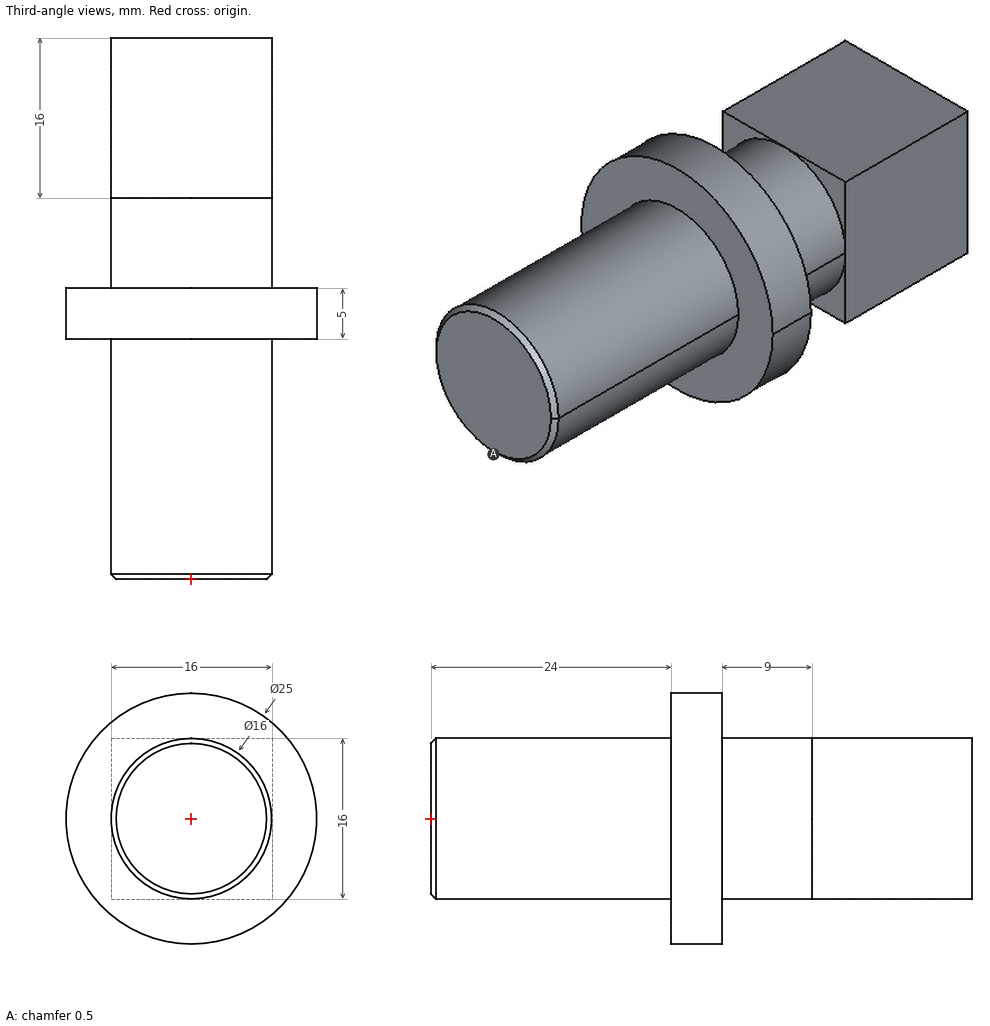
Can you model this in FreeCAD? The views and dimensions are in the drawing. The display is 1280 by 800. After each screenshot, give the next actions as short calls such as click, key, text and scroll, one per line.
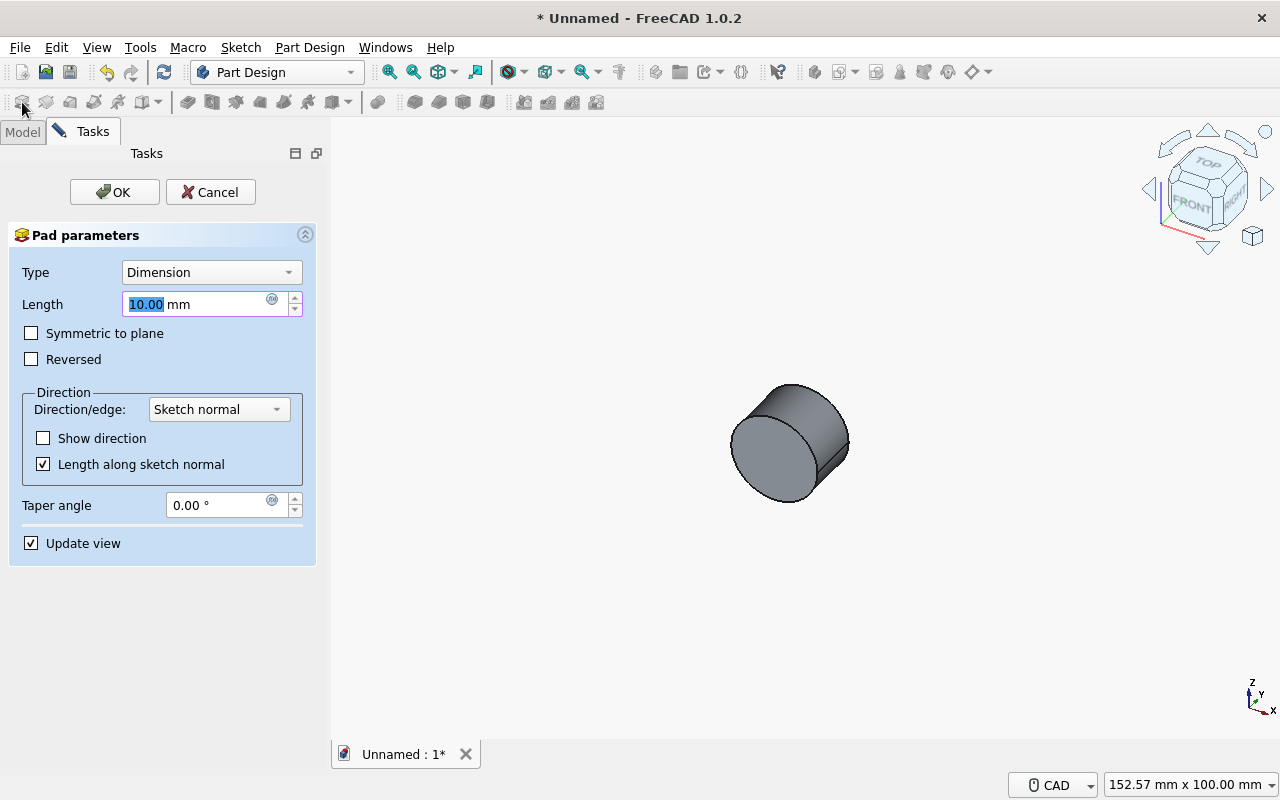
text(24)
key(Tab)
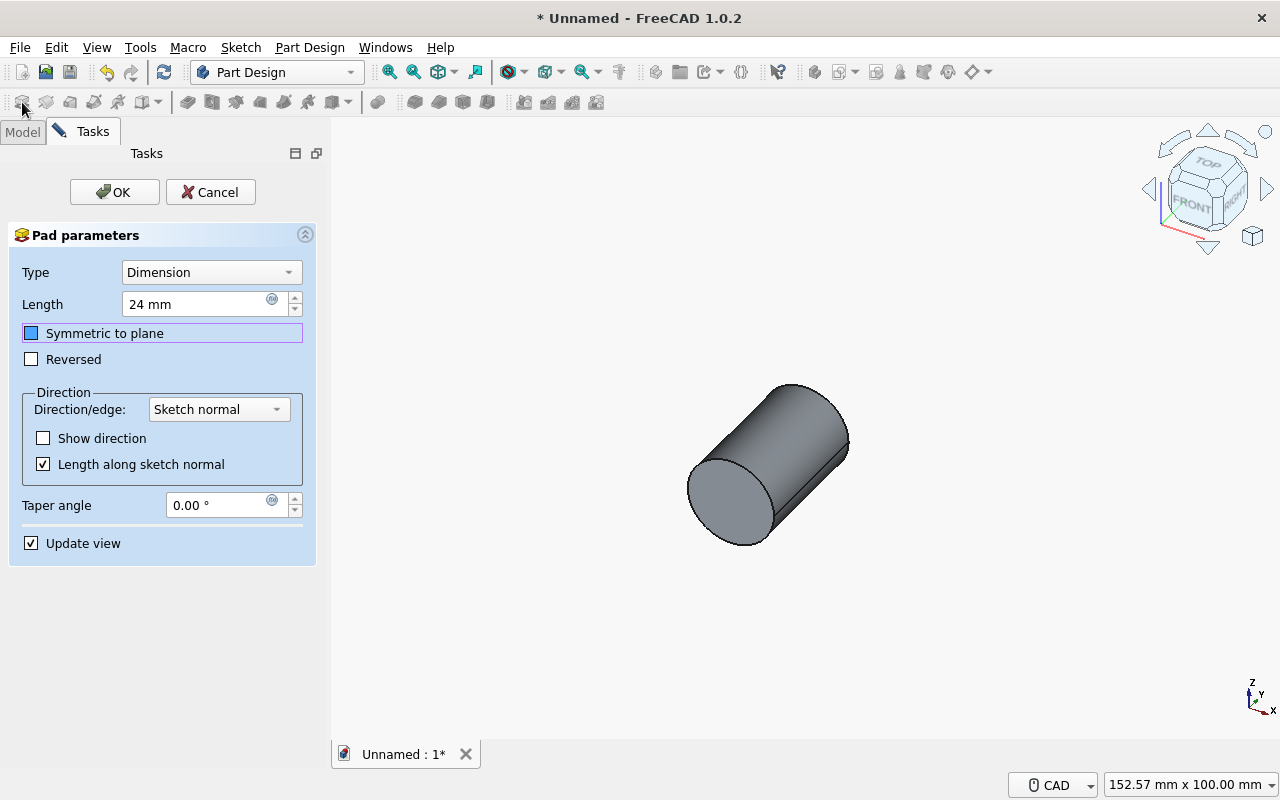
click(30, 359)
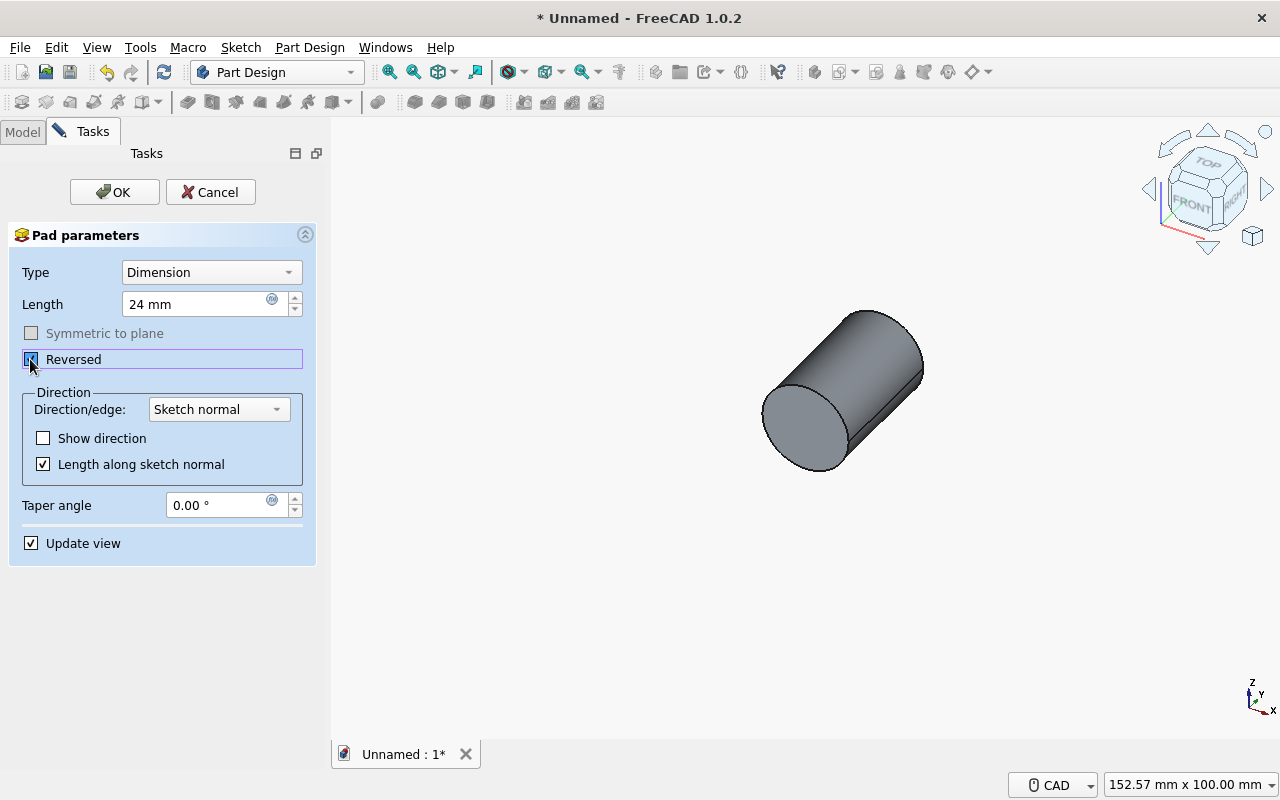
click(115, 192)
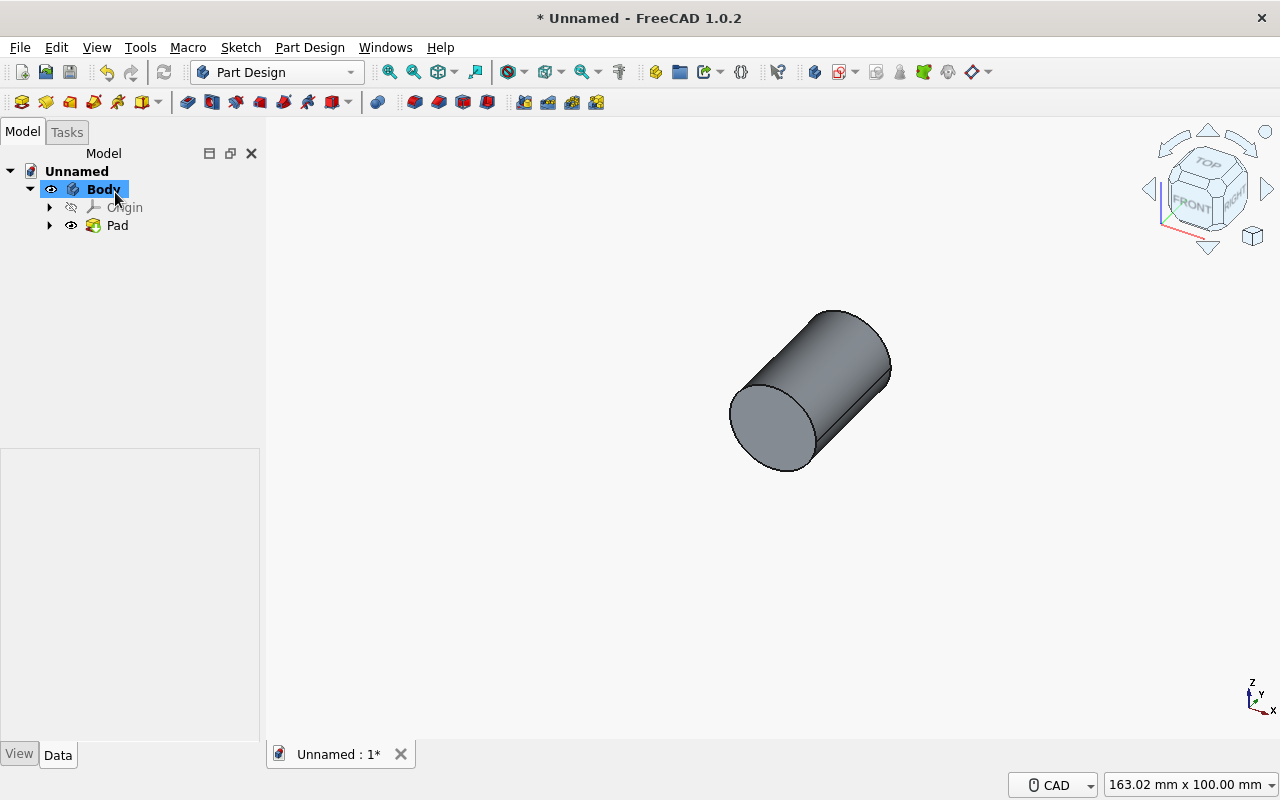
click(390, 72)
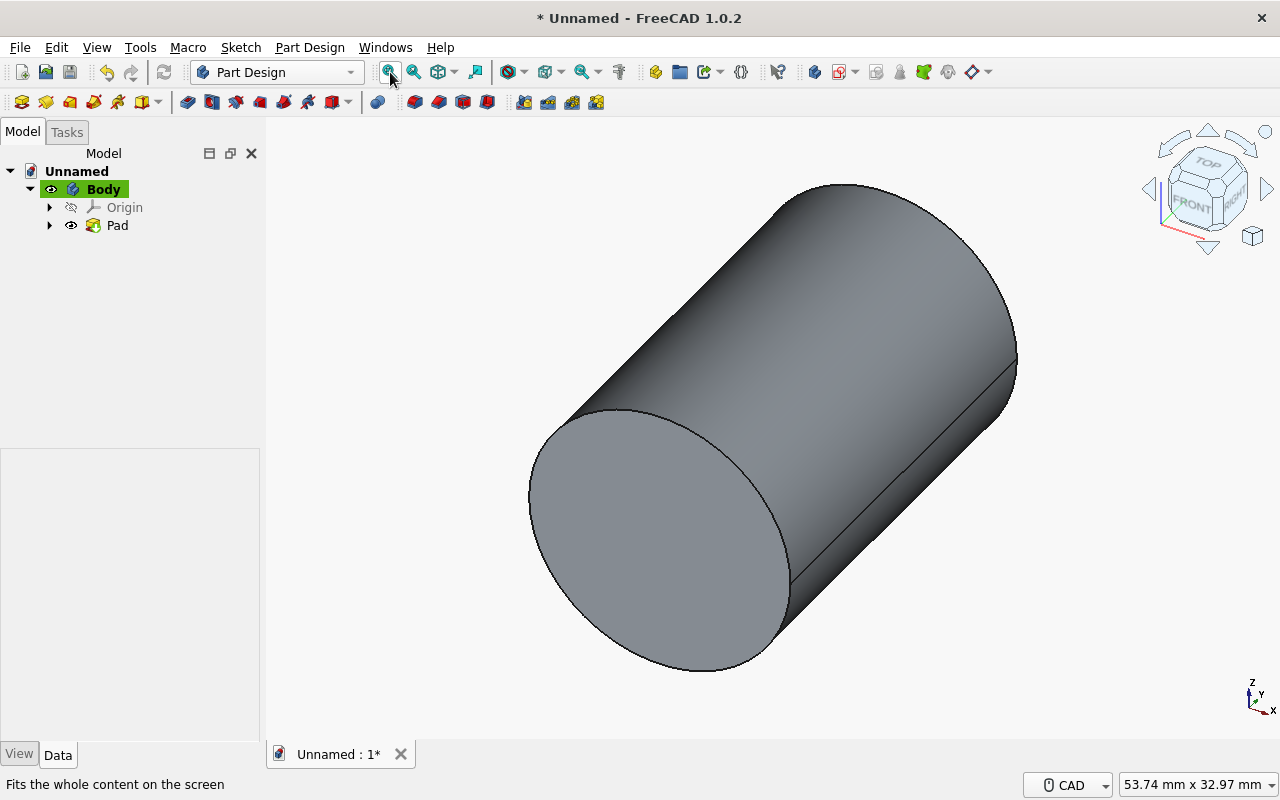
click(619, 408)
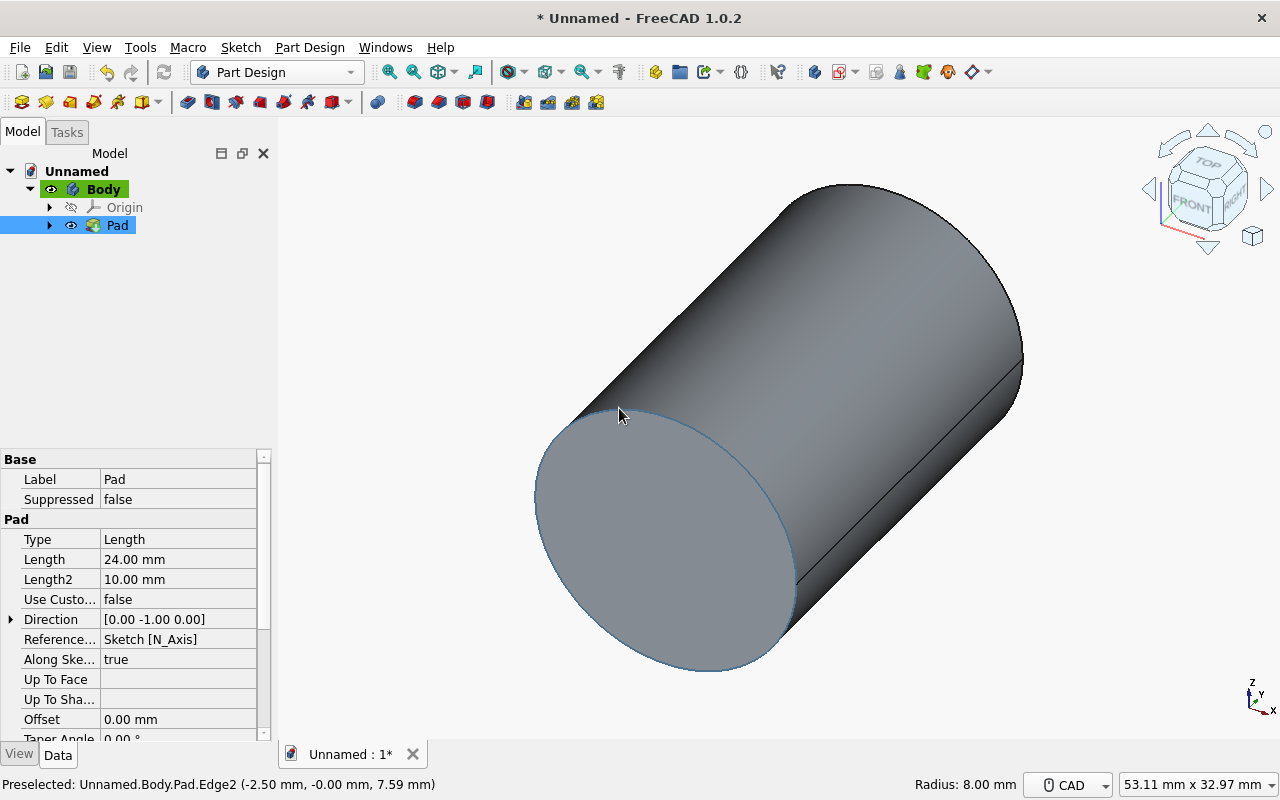
click(440, 102)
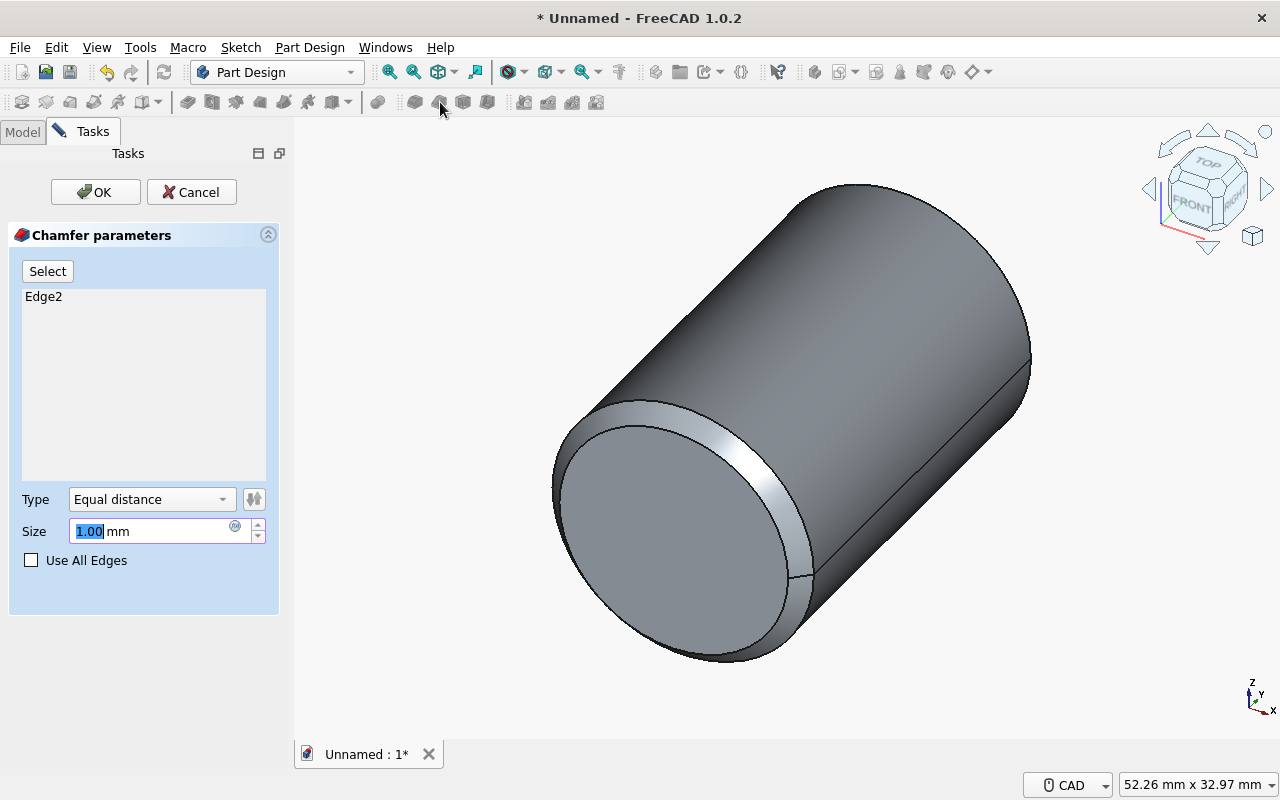
text(0.5)
key(Tab)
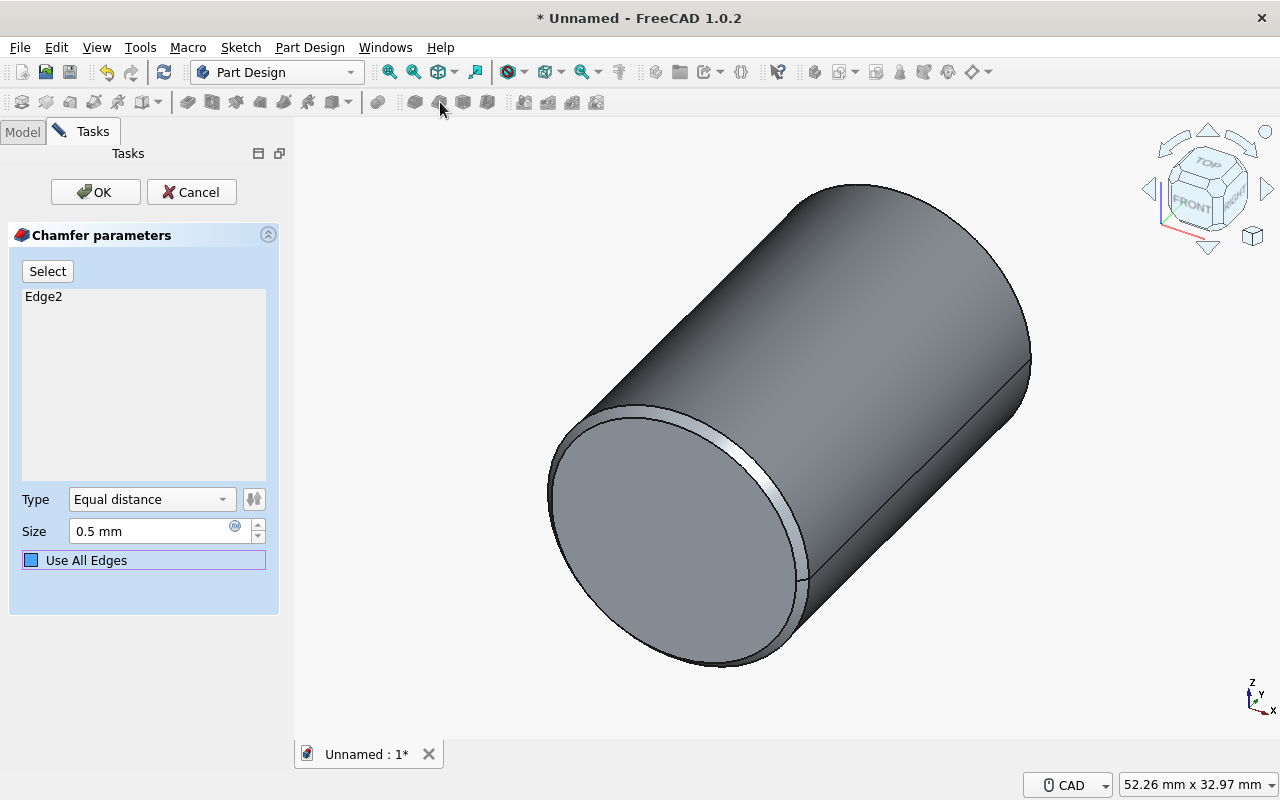
click(96, 192)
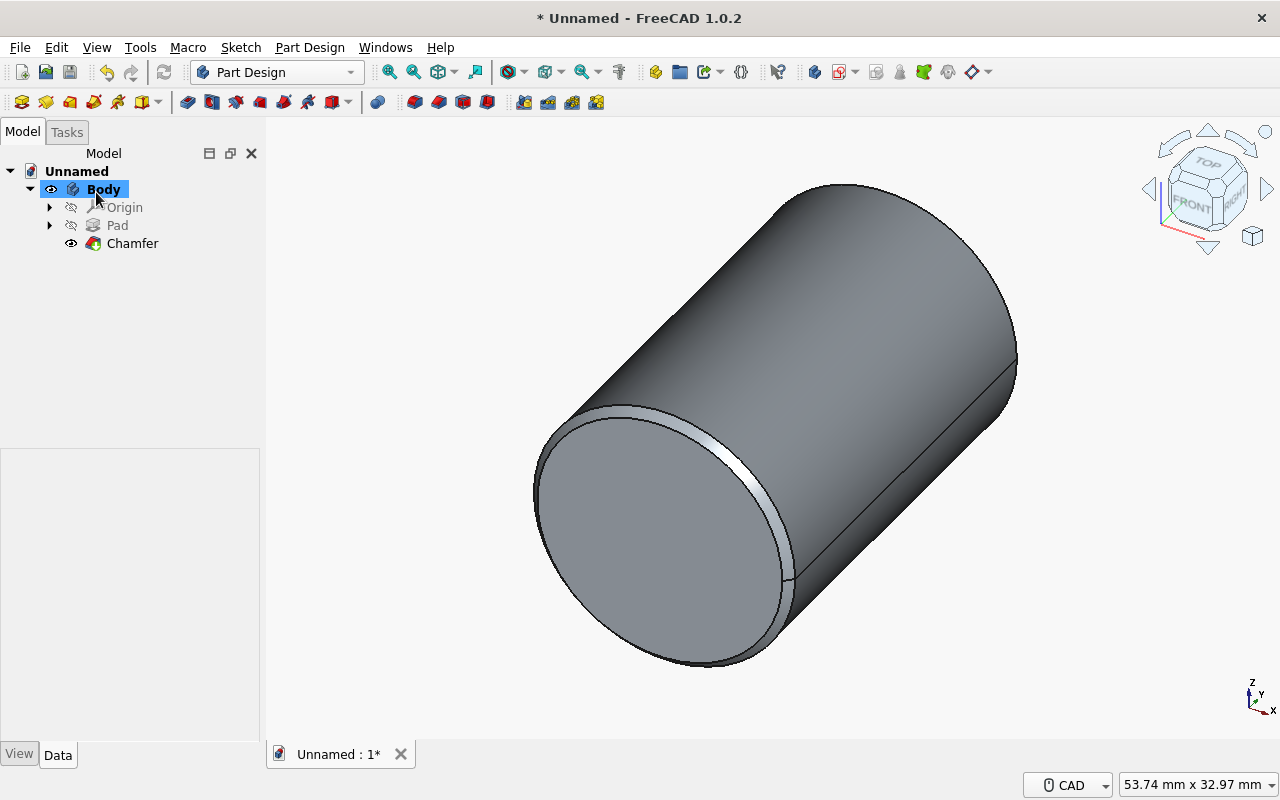
key(4)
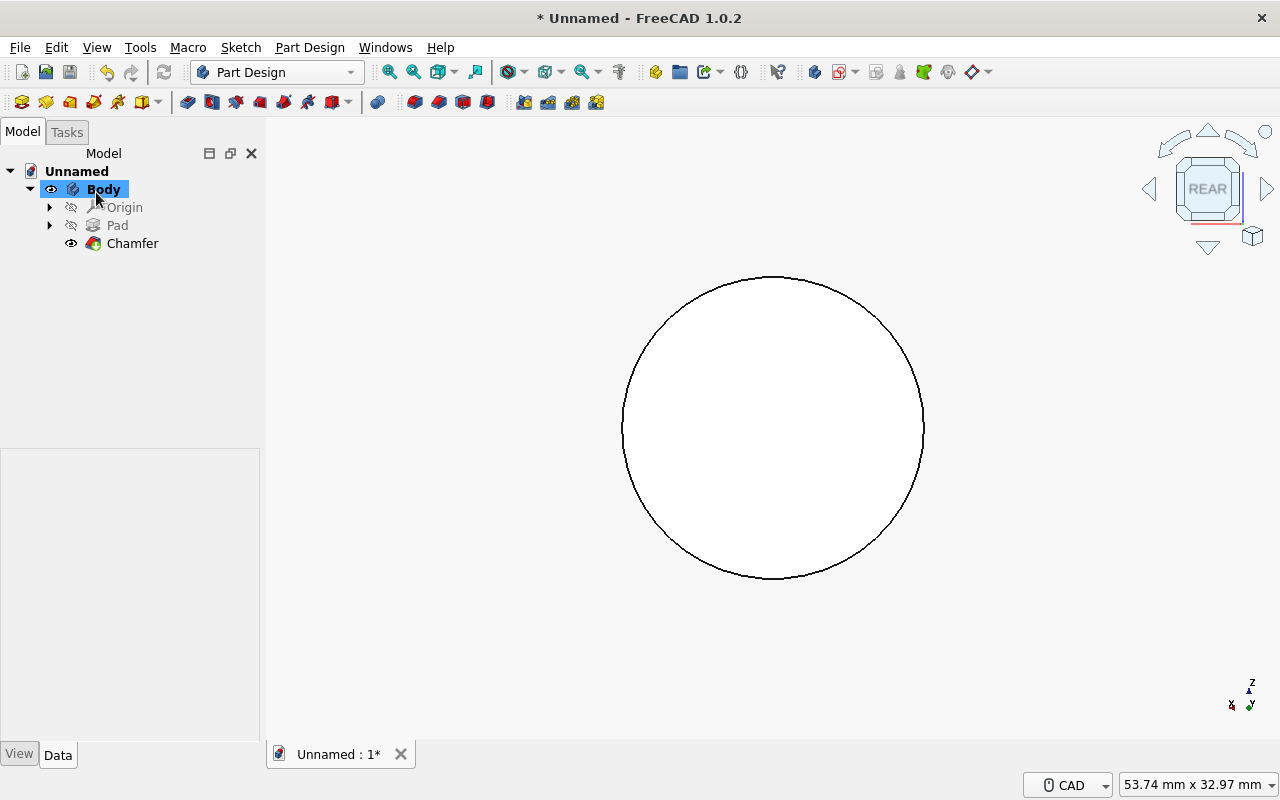
click(773, 427)